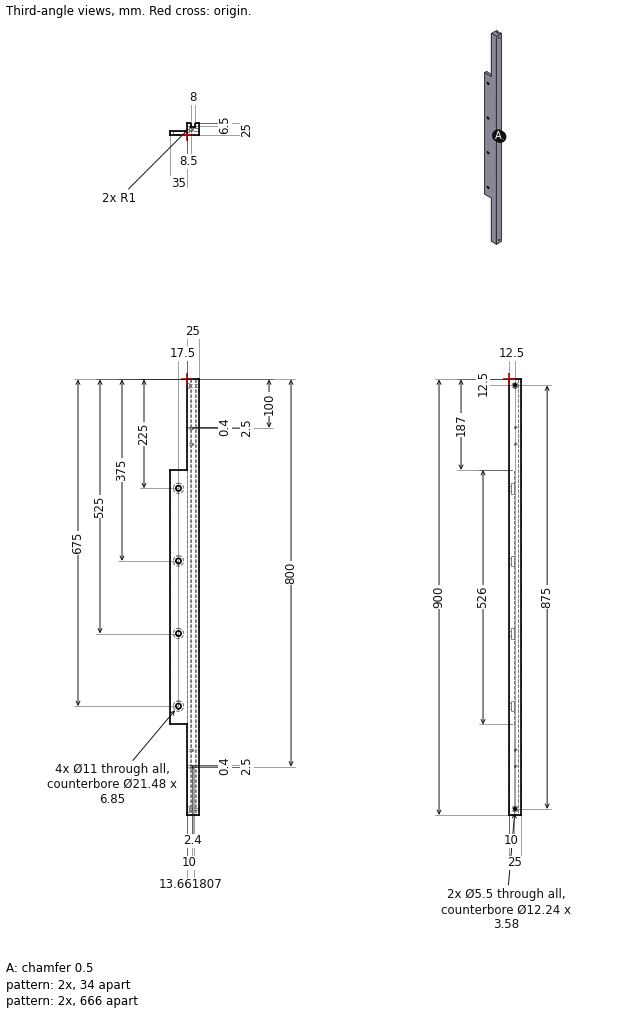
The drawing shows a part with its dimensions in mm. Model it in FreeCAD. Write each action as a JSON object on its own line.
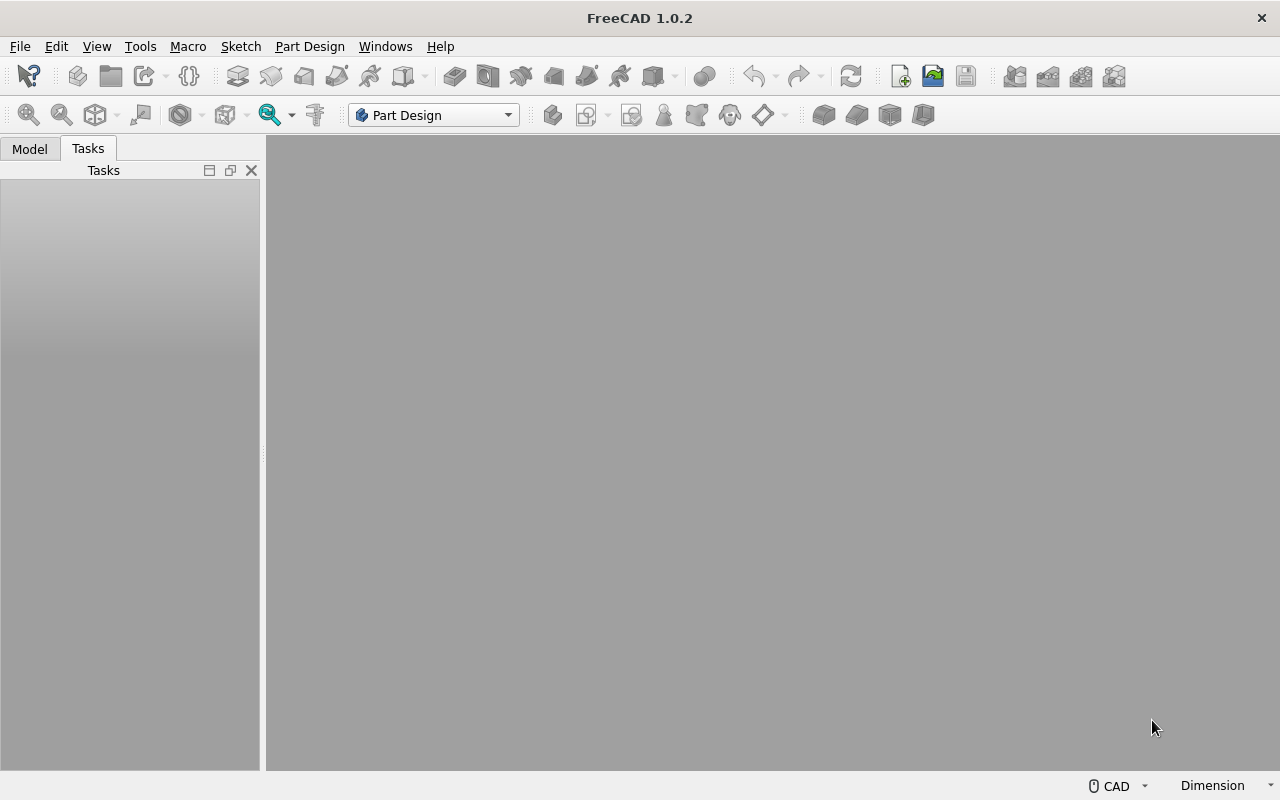
{"action": "key", "text": "ctrl+n"}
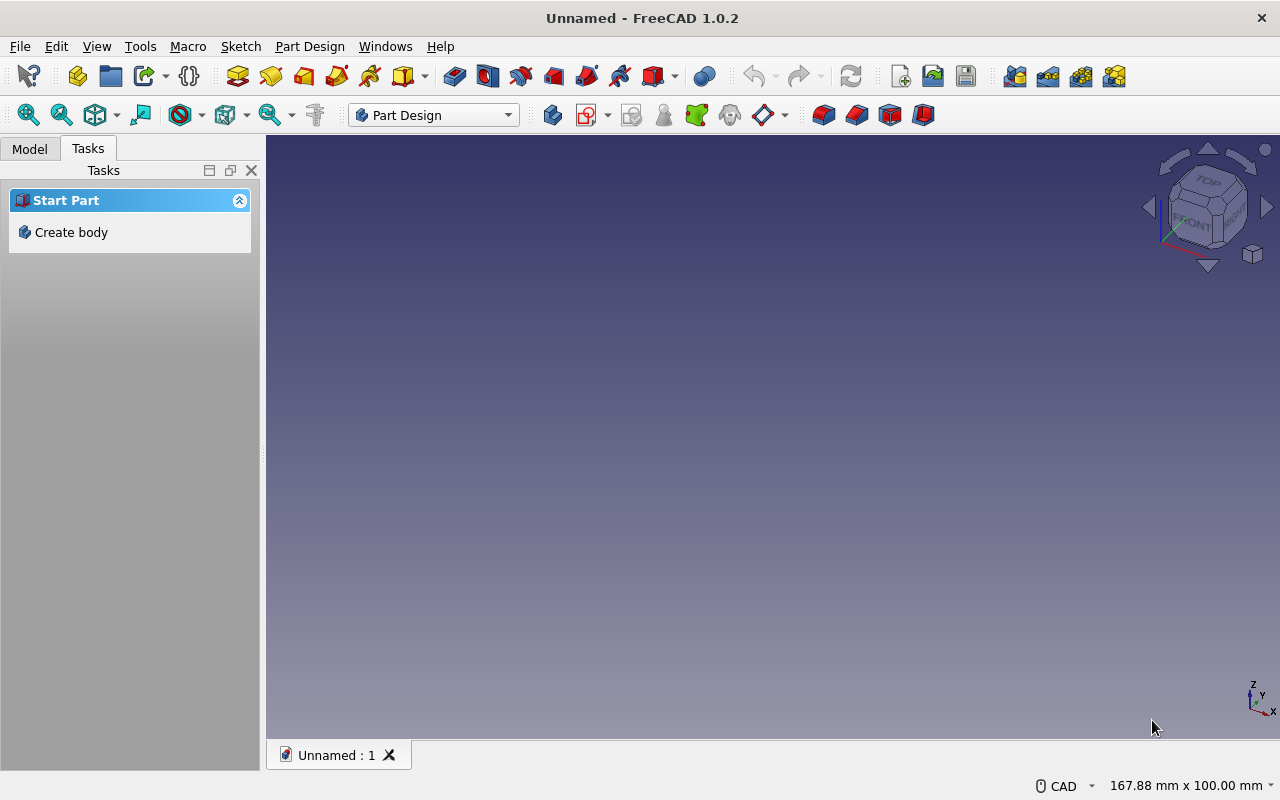
{"action": "left_click", "coordinate": [586, 116]}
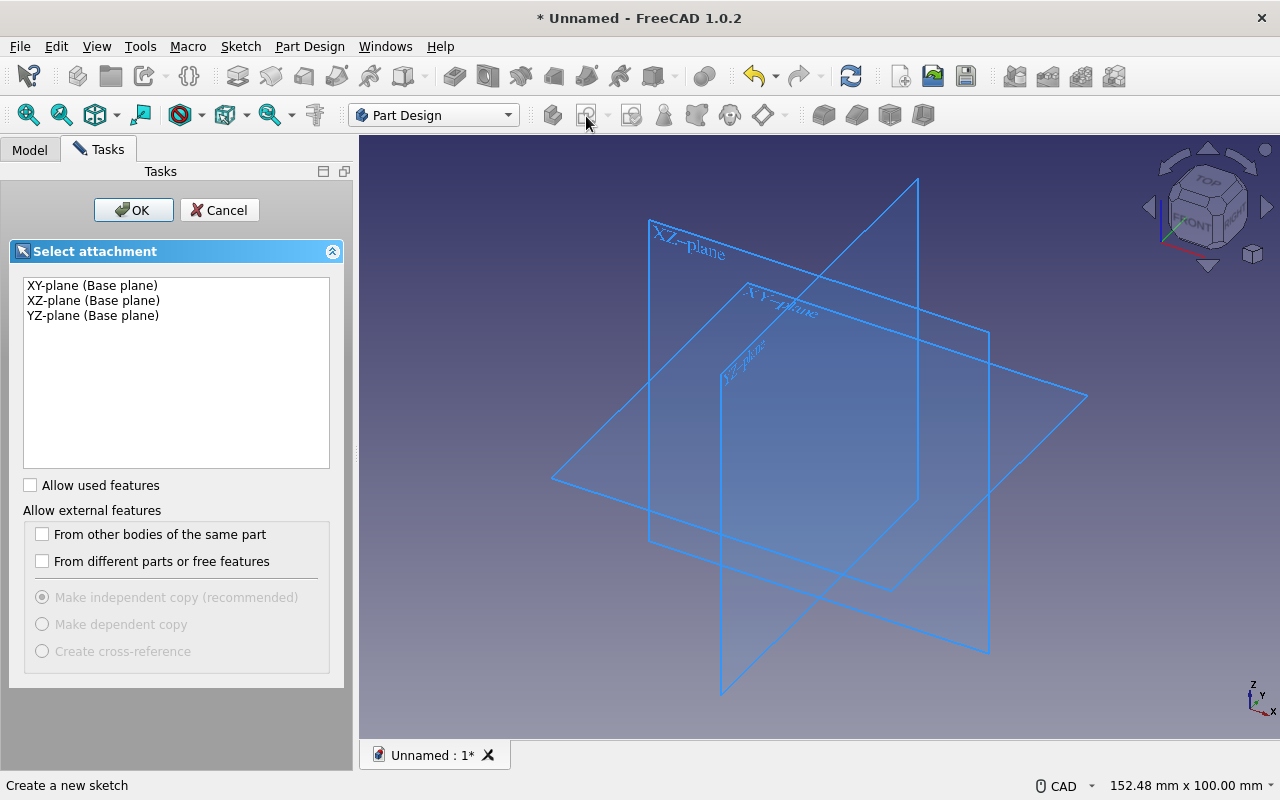
{"action": "left_click", "coordinate": [84, 316]}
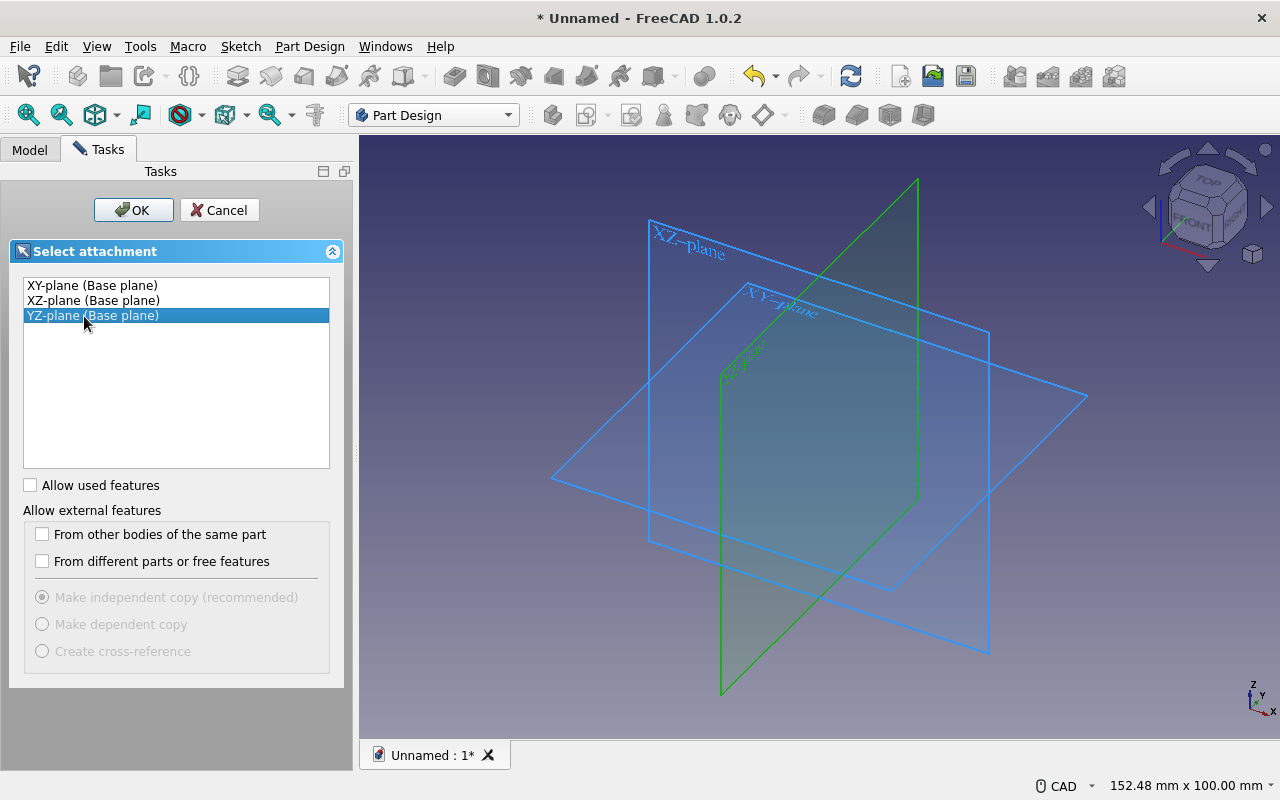
{"action": "left_click", "coordinate": [134, 210]}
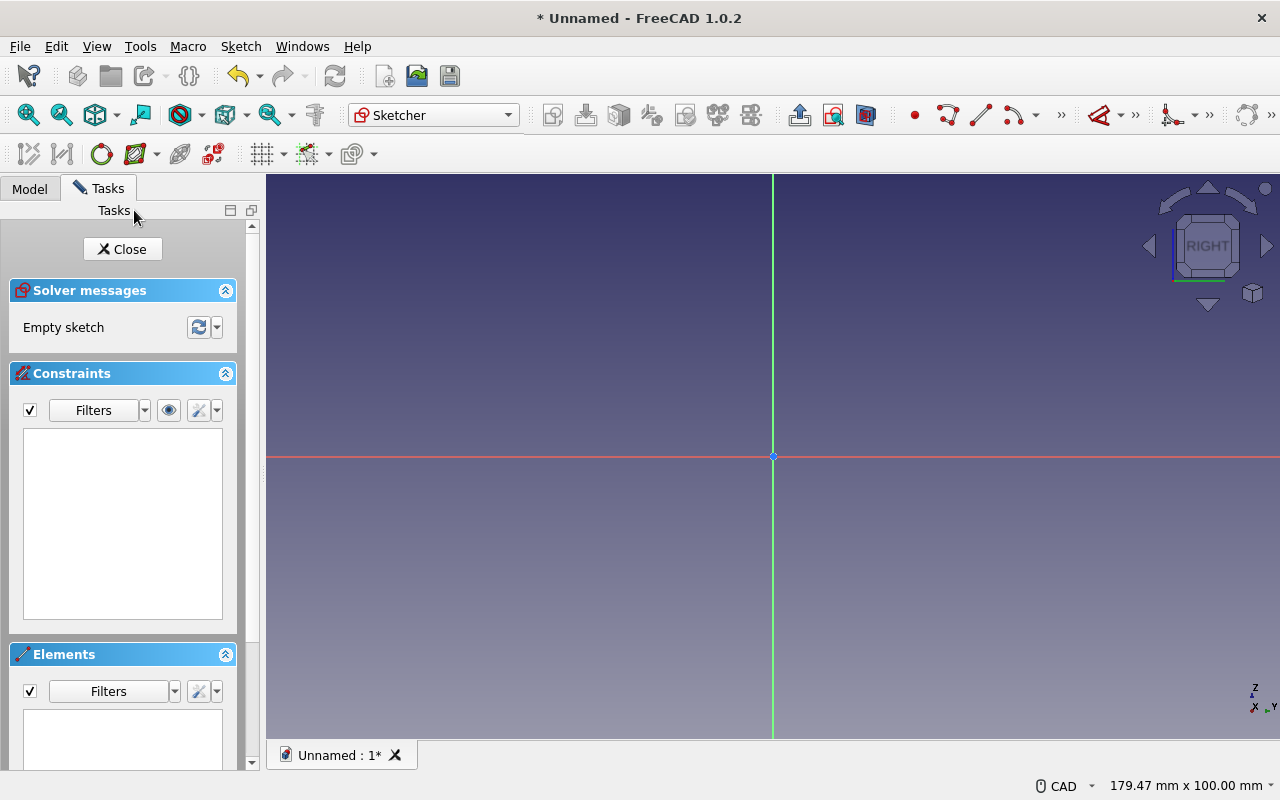
{"action": "scroll", "coordinate": [693, 253], "scroll_direction": "down", "scroll_amount": 13}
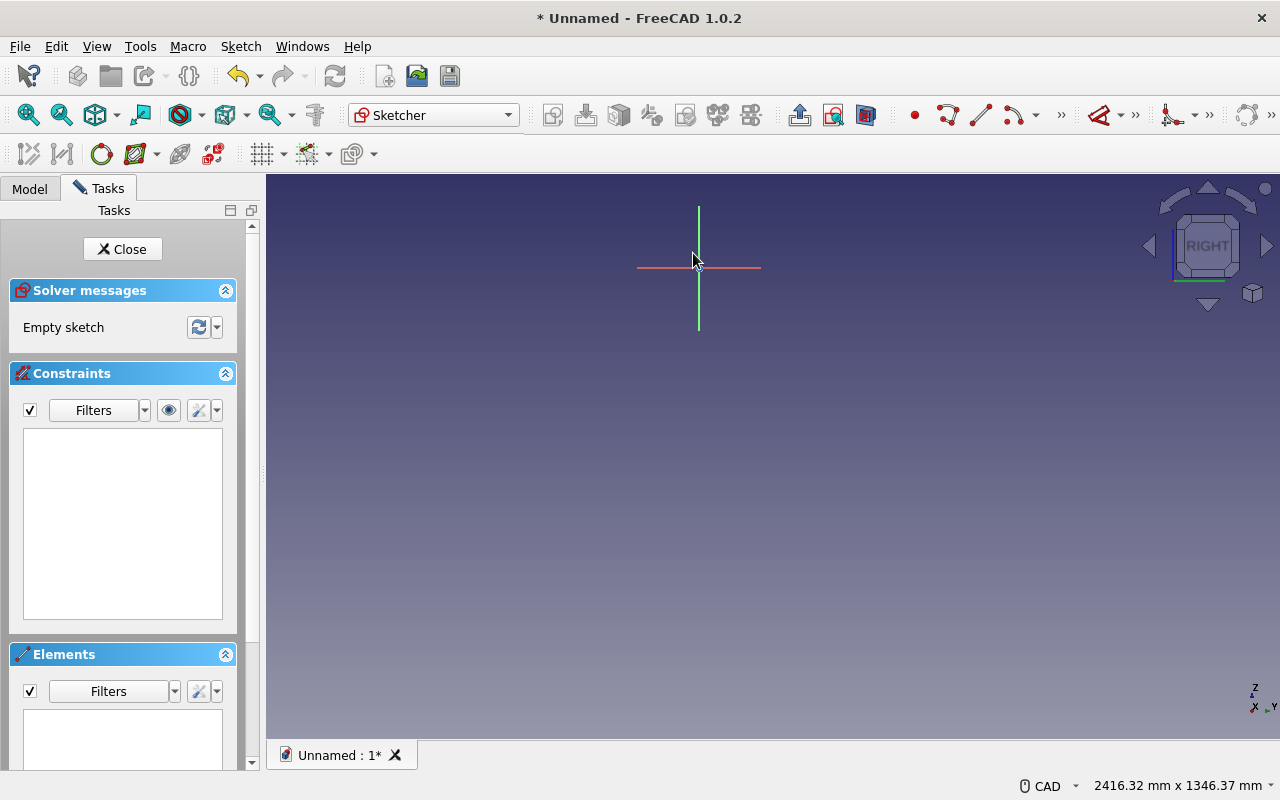
{"action": "key", "text": "g r"}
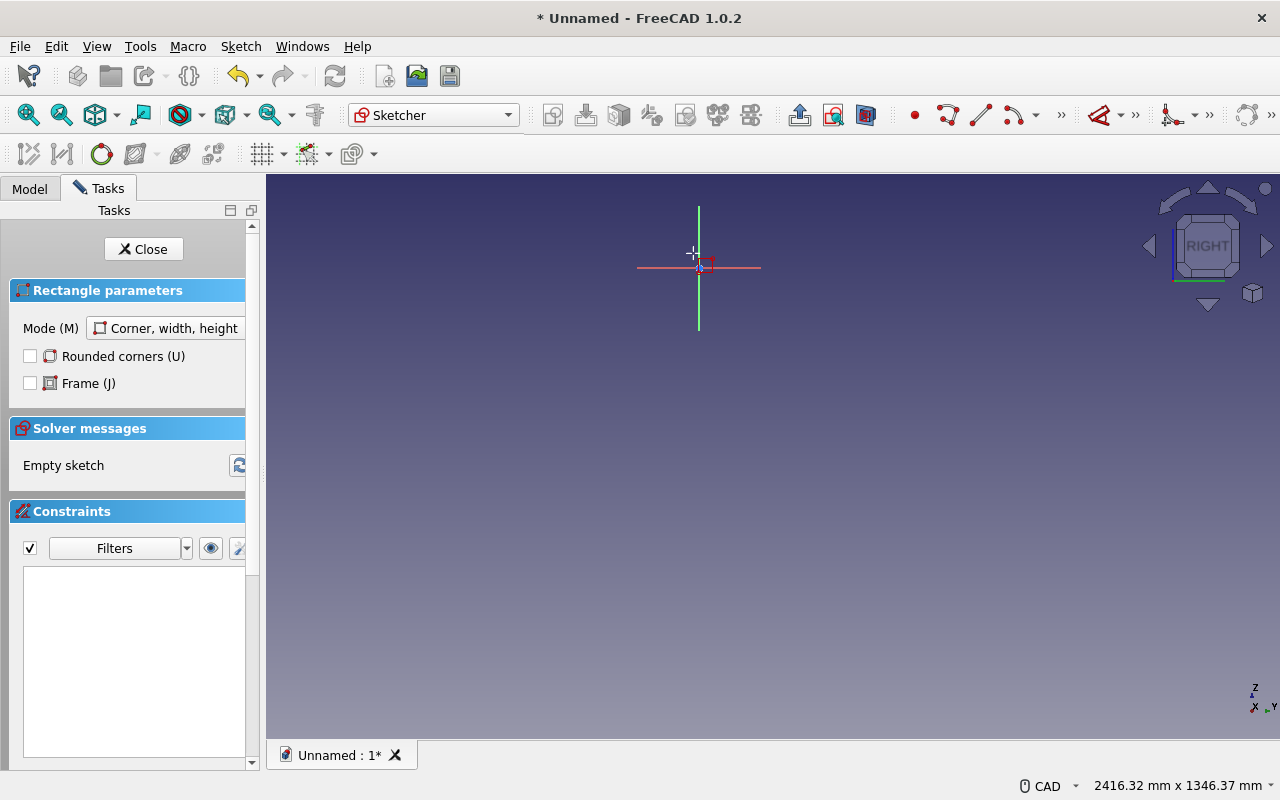
{"action": "scroll", "coordinate": [699, 268], "scroll_direction": "up", "scroll_amount": 3}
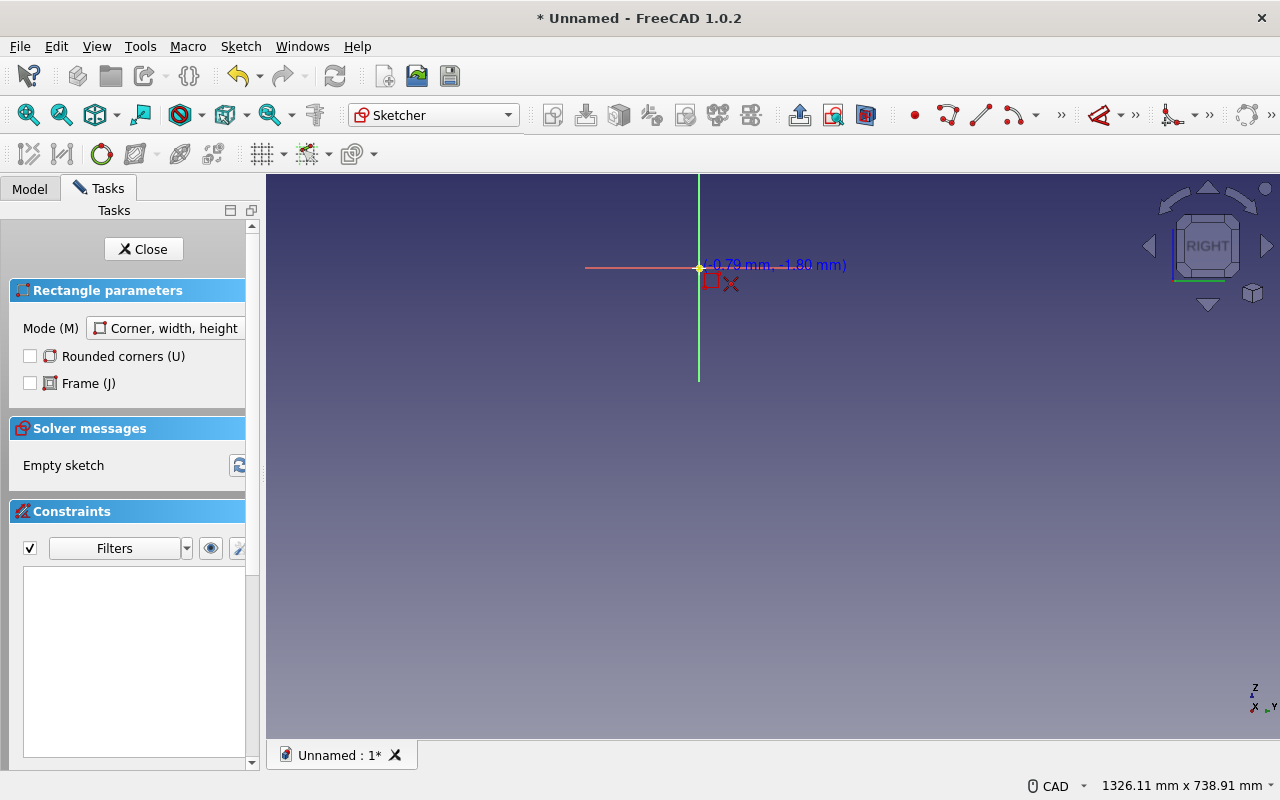
{"action": "left_click", "coordinate": [699, 268]}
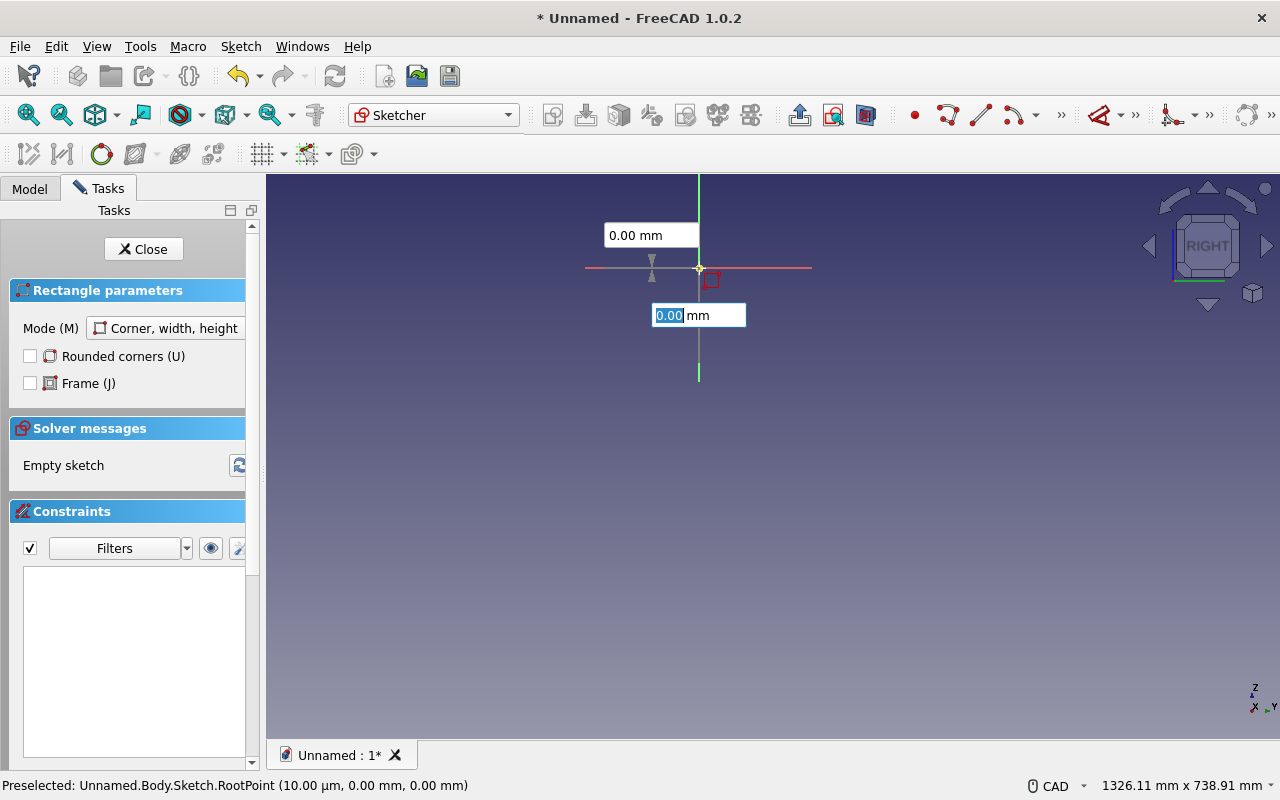
{"action": "scroll", "coordinate": [699, 267], "scroll_direction": "down", "scroll_amount": 3}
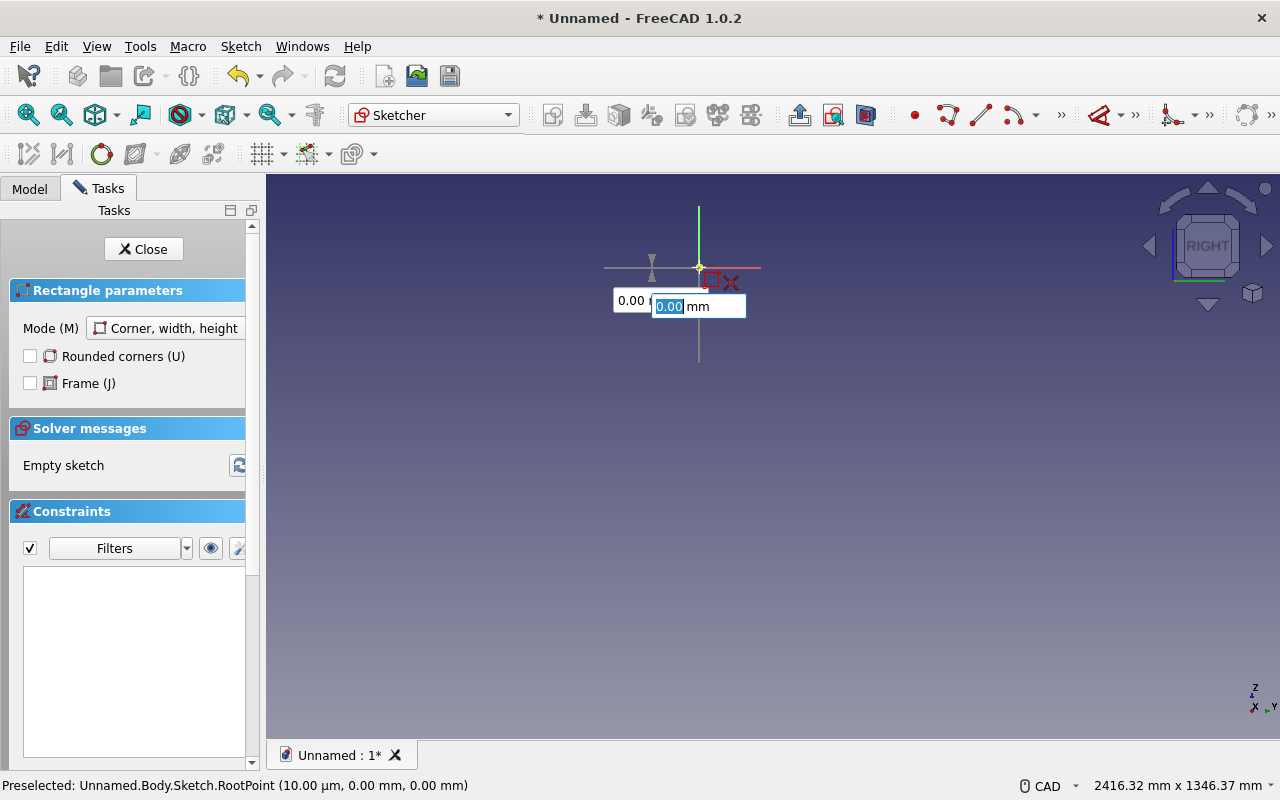
{"action": "scroll", "coordinate": [710, 645], "scroll_direction": "up", "scroll_amount": 3}